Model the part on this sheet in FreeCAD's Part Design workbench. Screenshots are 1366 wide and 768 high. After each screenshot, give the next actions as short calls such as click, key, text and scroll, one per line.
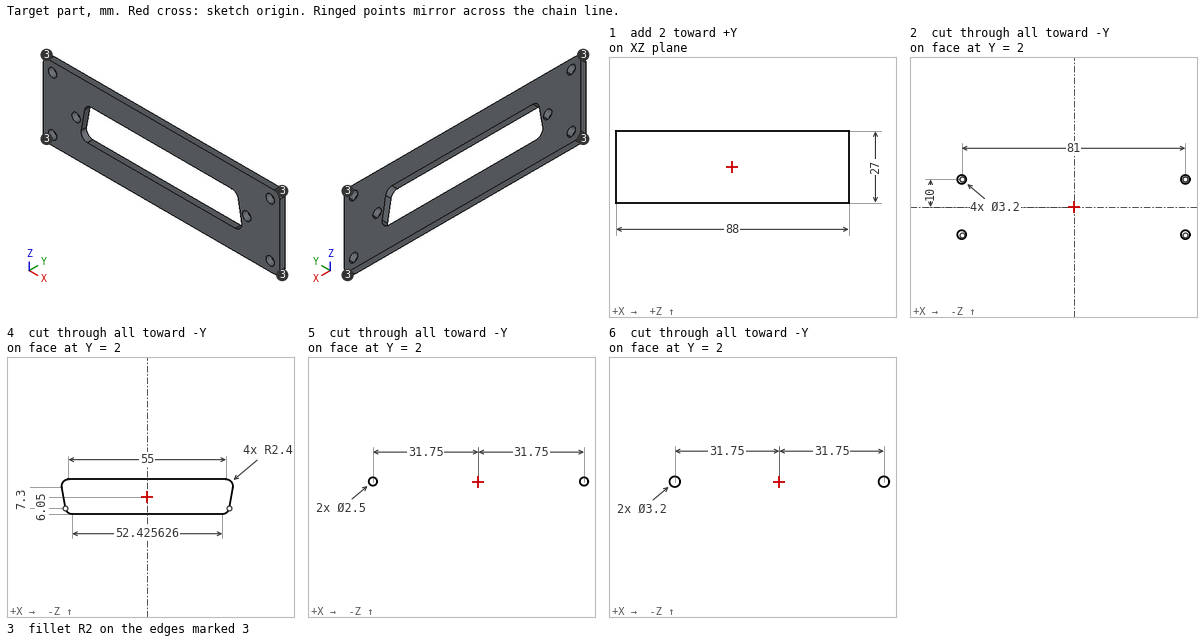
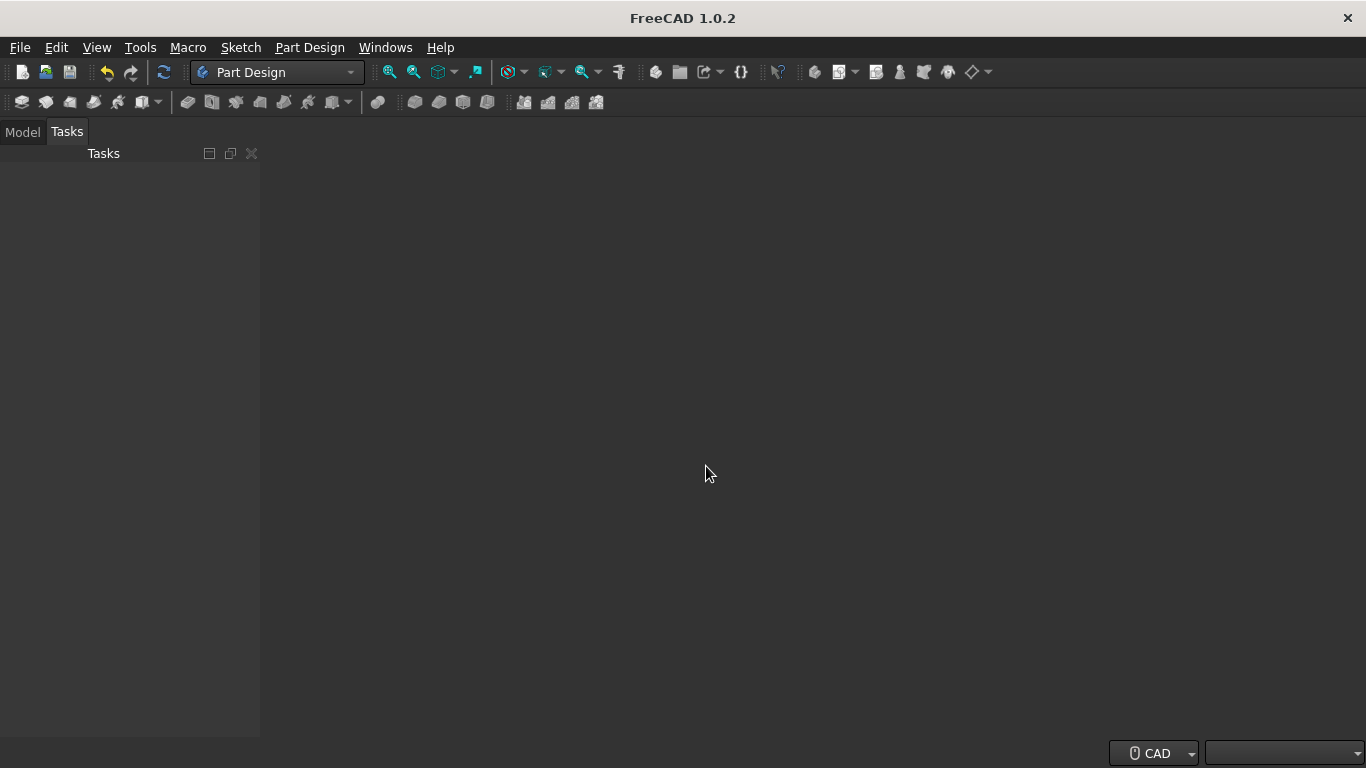
click(22, 72)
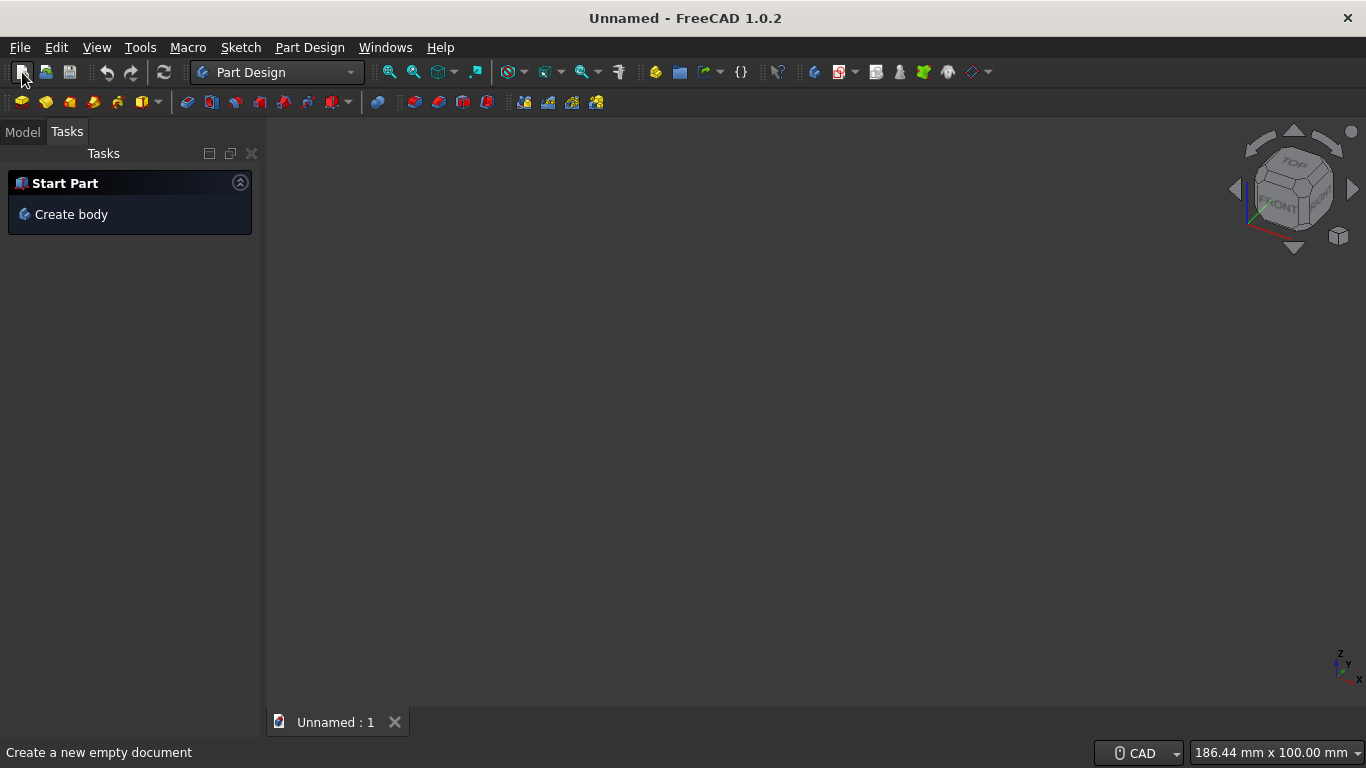
click(840, 72)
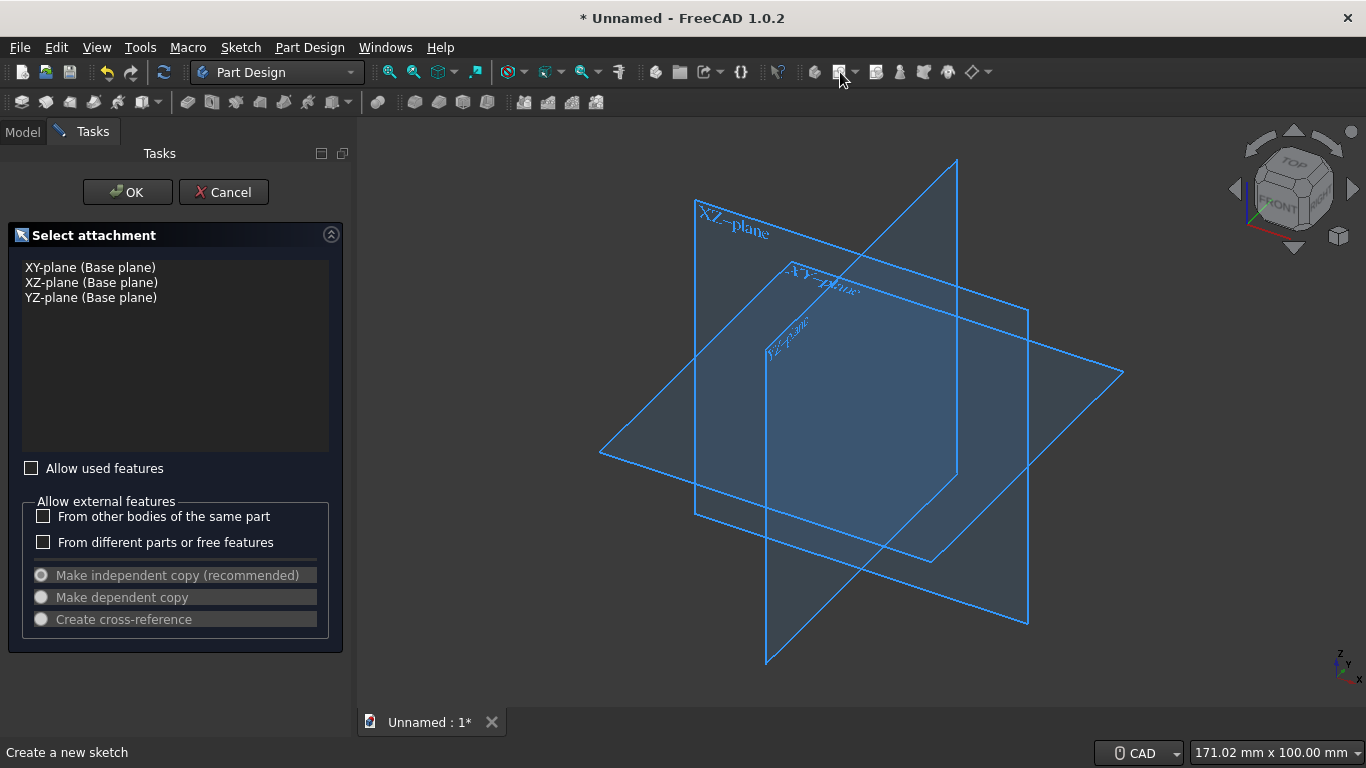
click(82, 282)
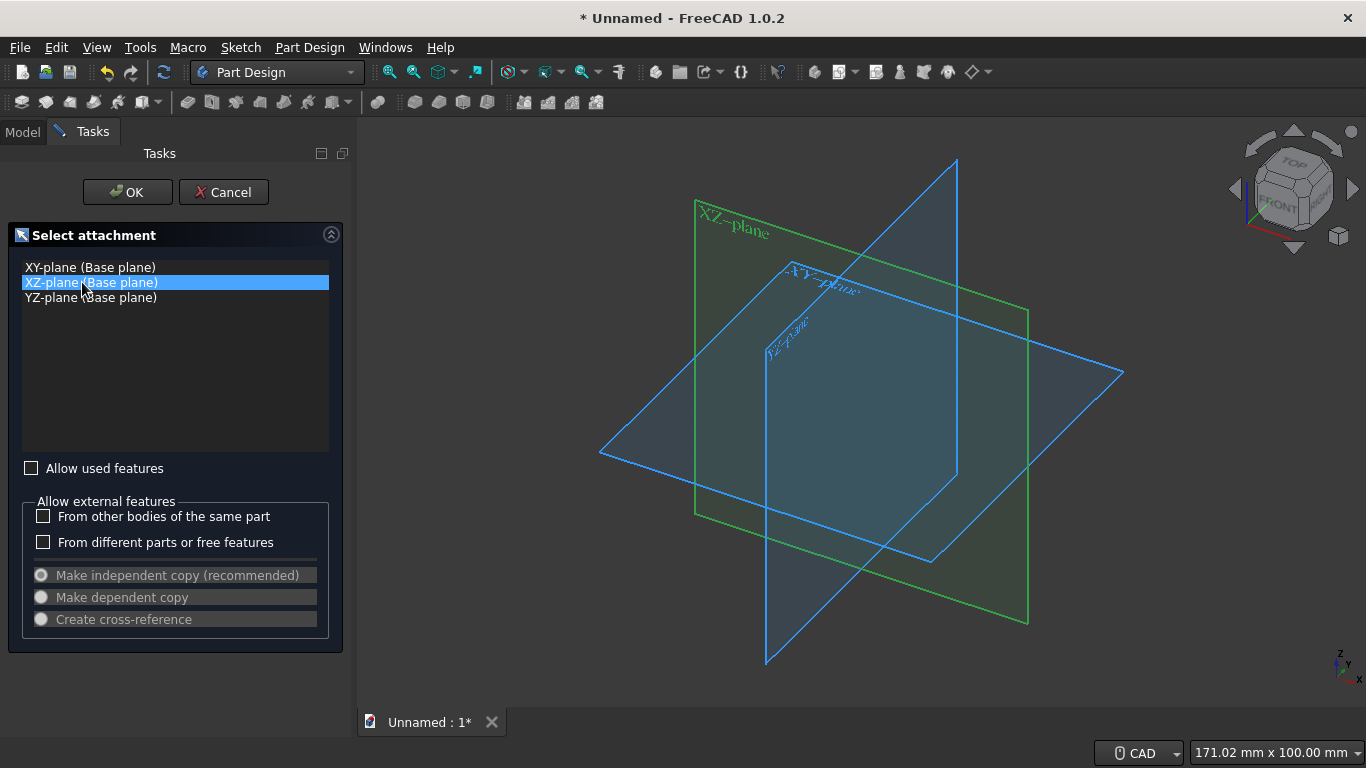
click(128, 192)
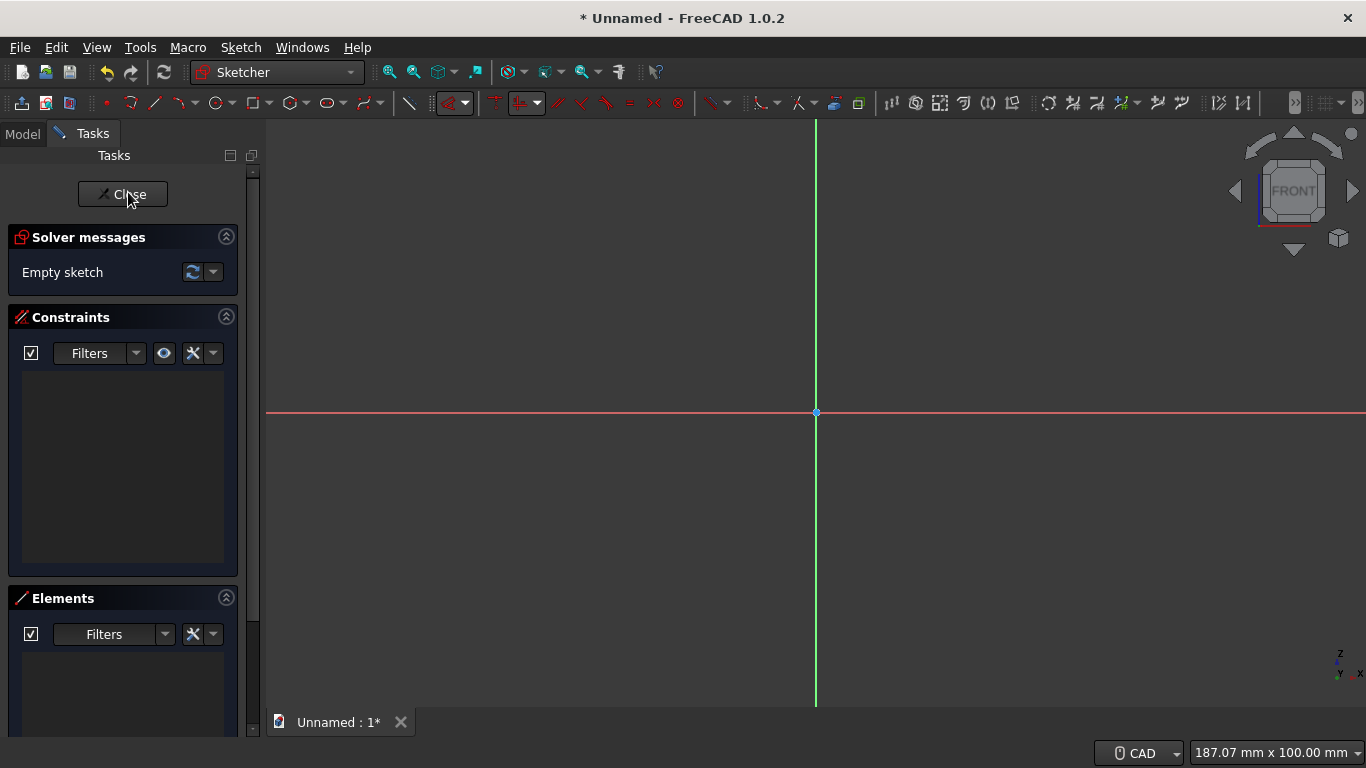
click(272, 104)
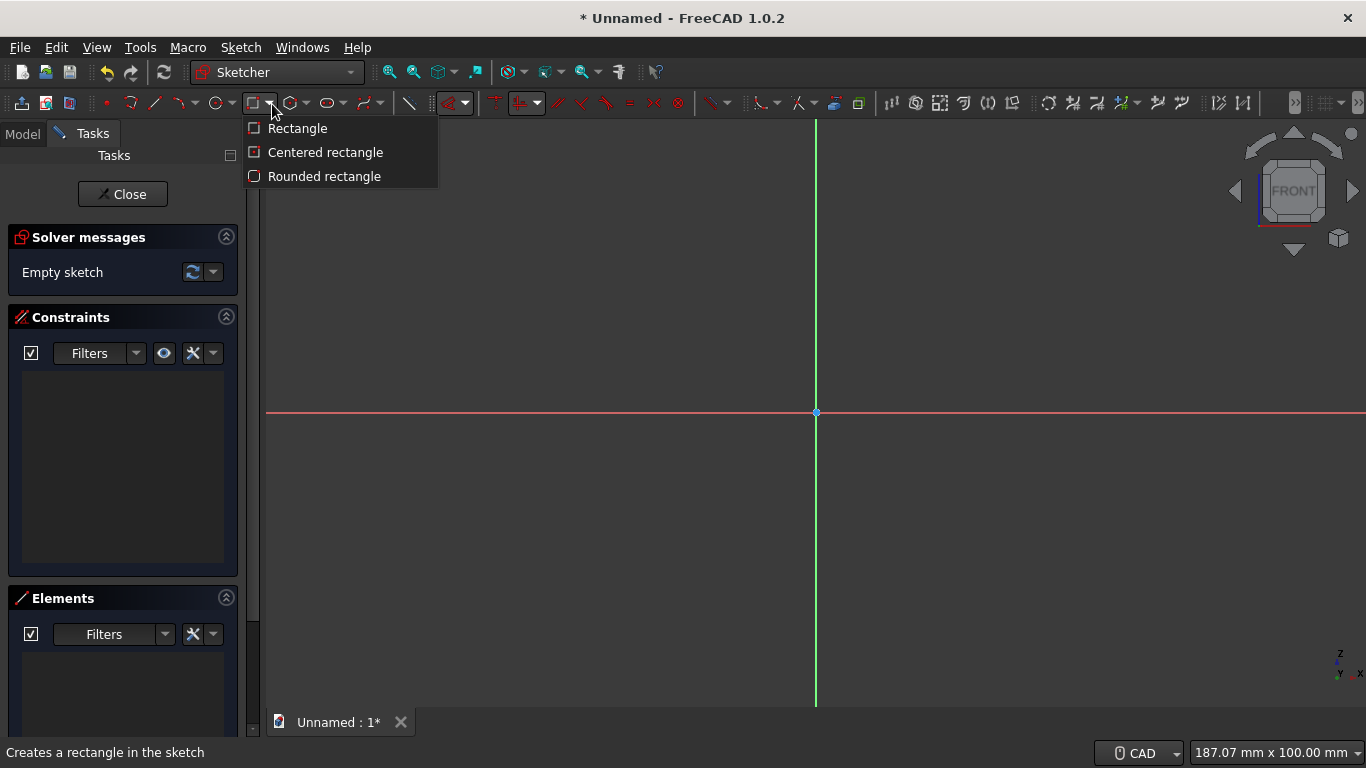
click(340, 152)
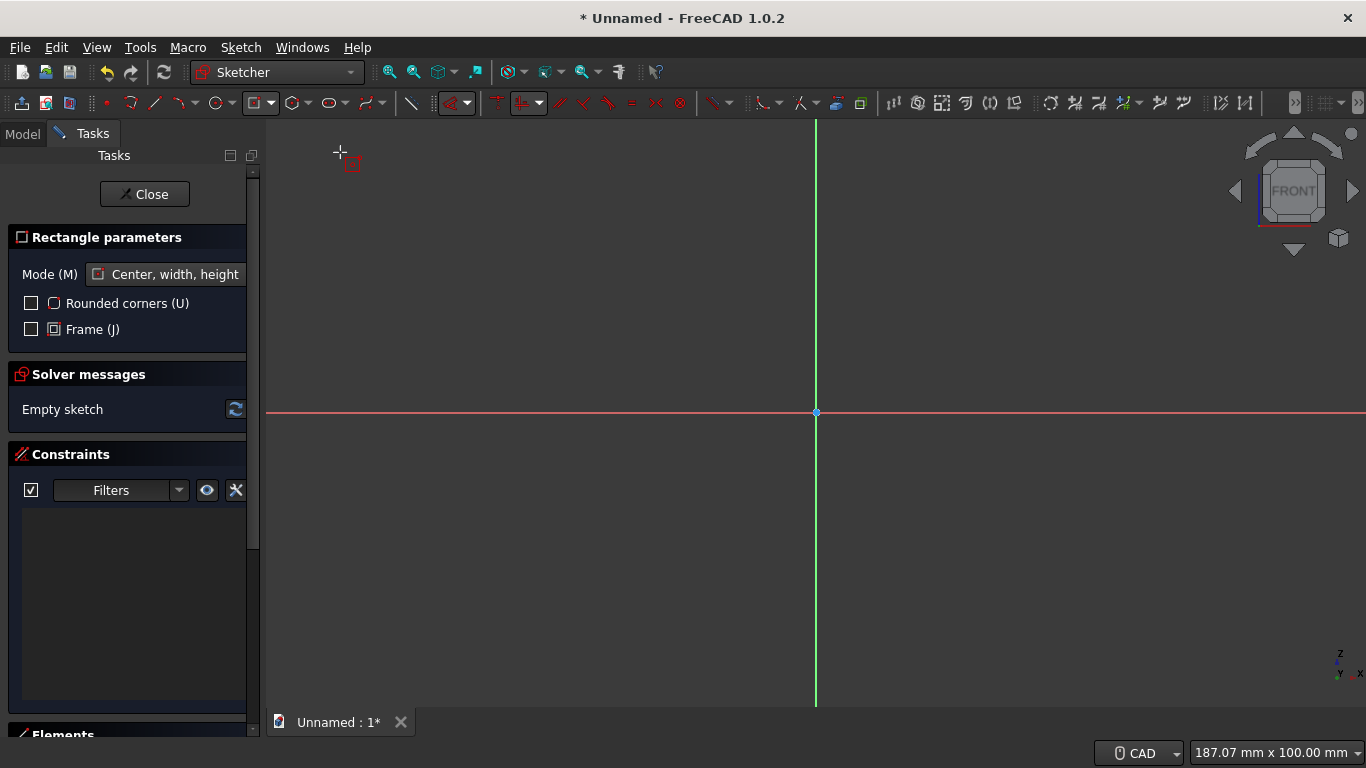
click(816, 413)
click(1075, 334)
key(Escape)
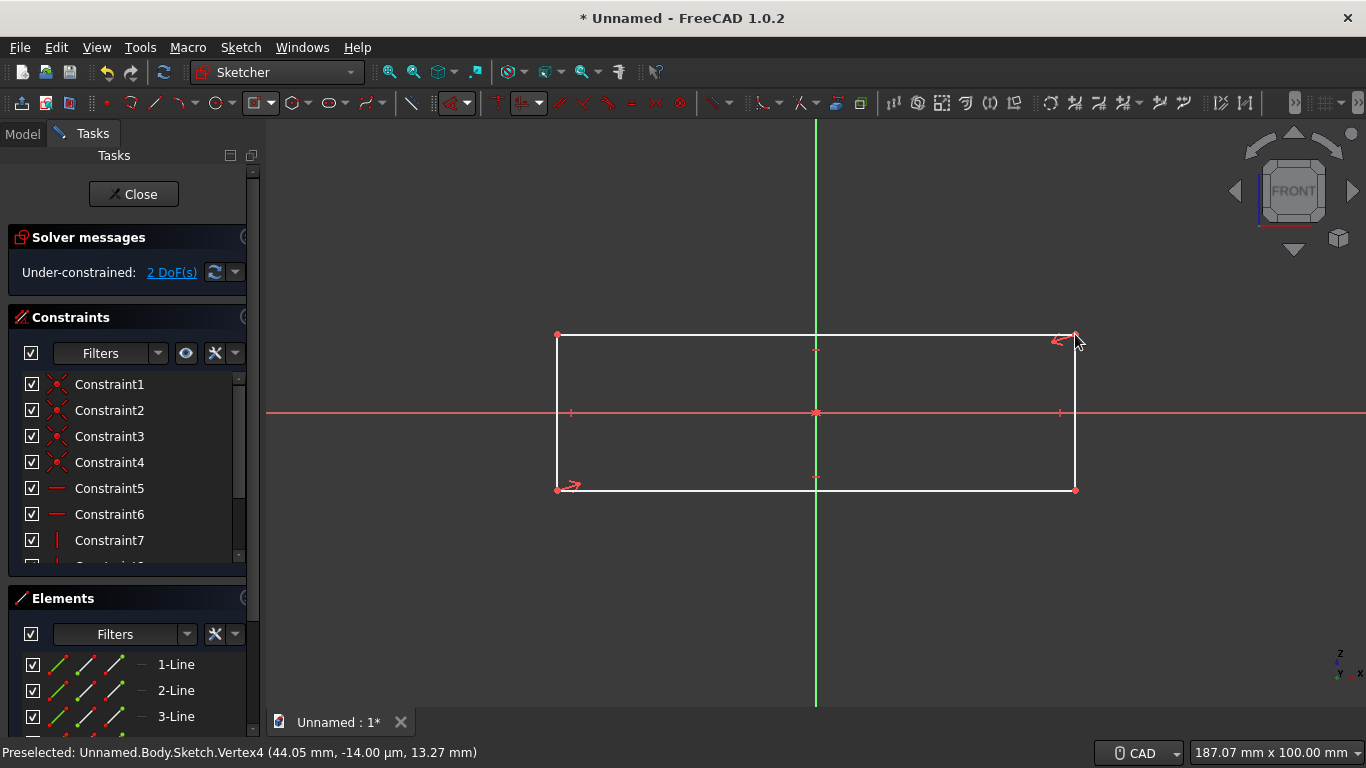
click(712, 491)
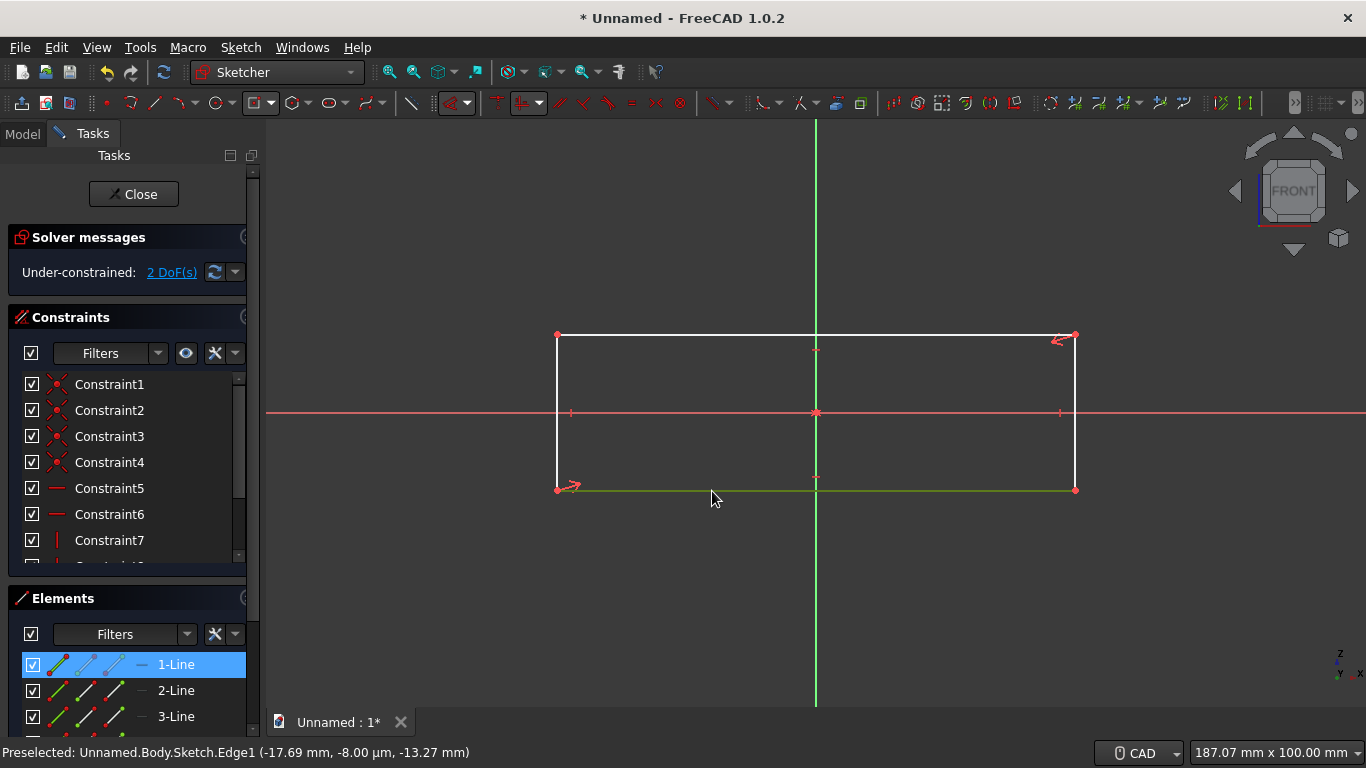
key(l)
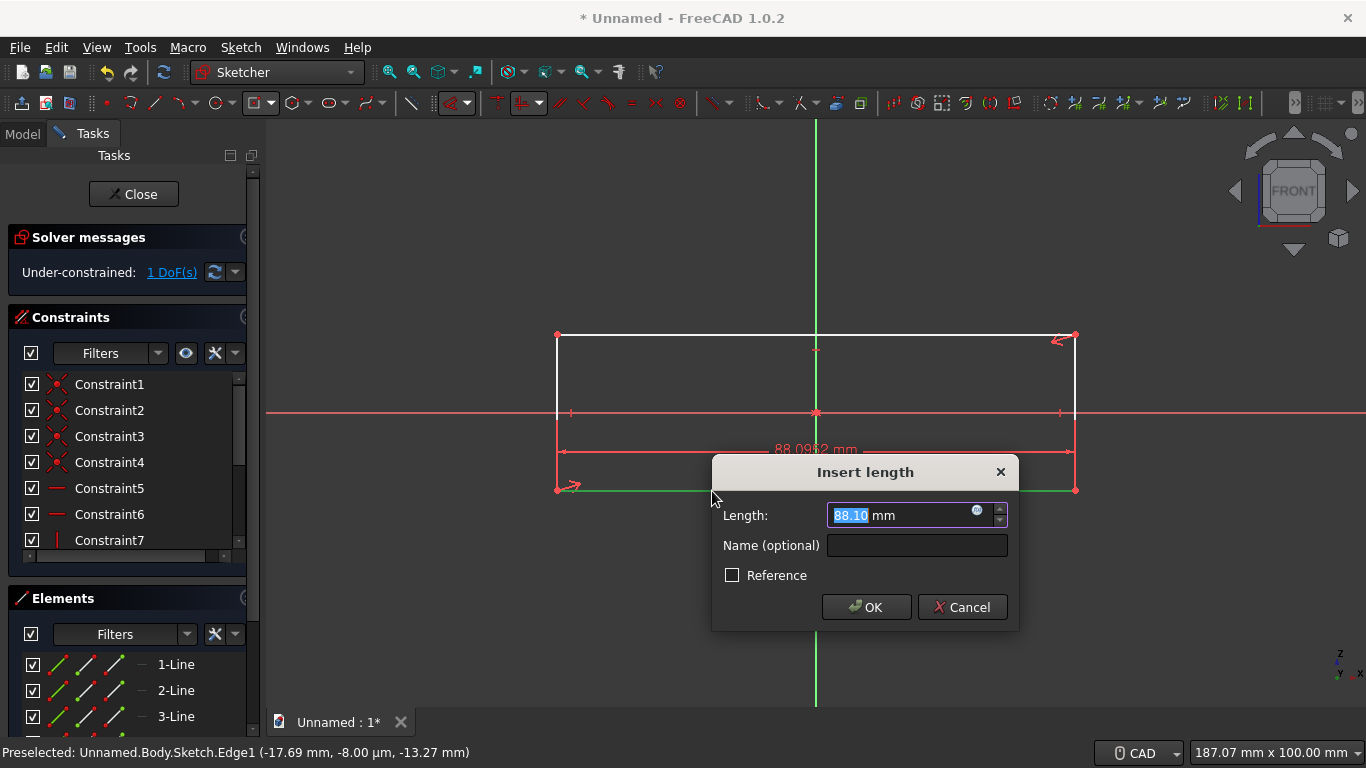
text(88)
key(Return)